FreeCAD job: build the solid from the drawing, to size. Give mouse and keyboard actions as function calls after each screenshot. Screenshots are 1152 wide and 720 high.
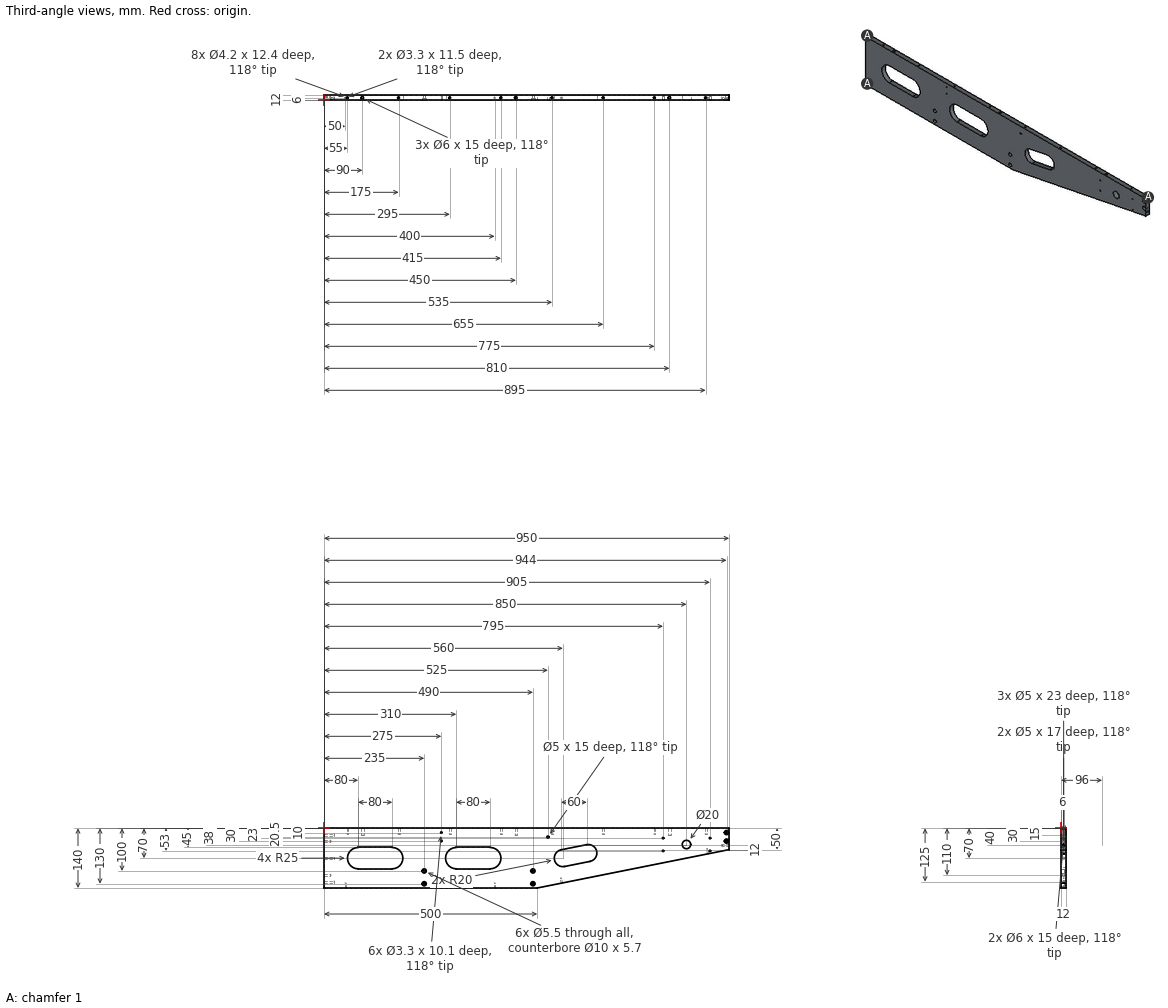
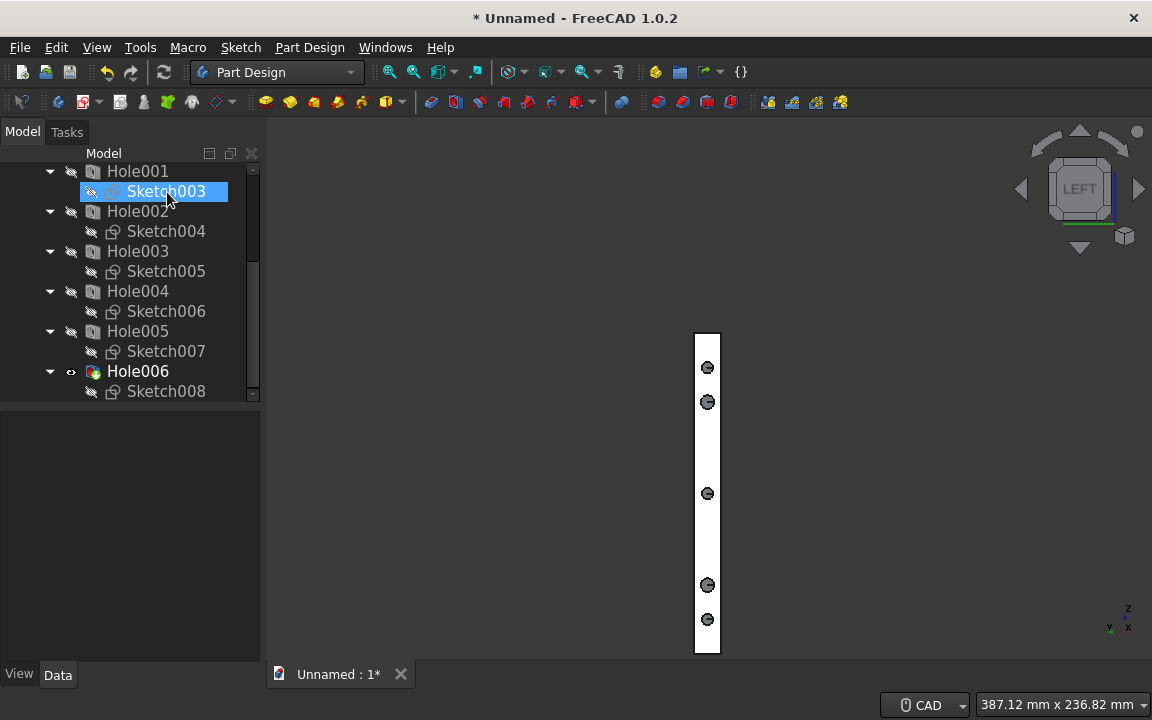
click(84, 102)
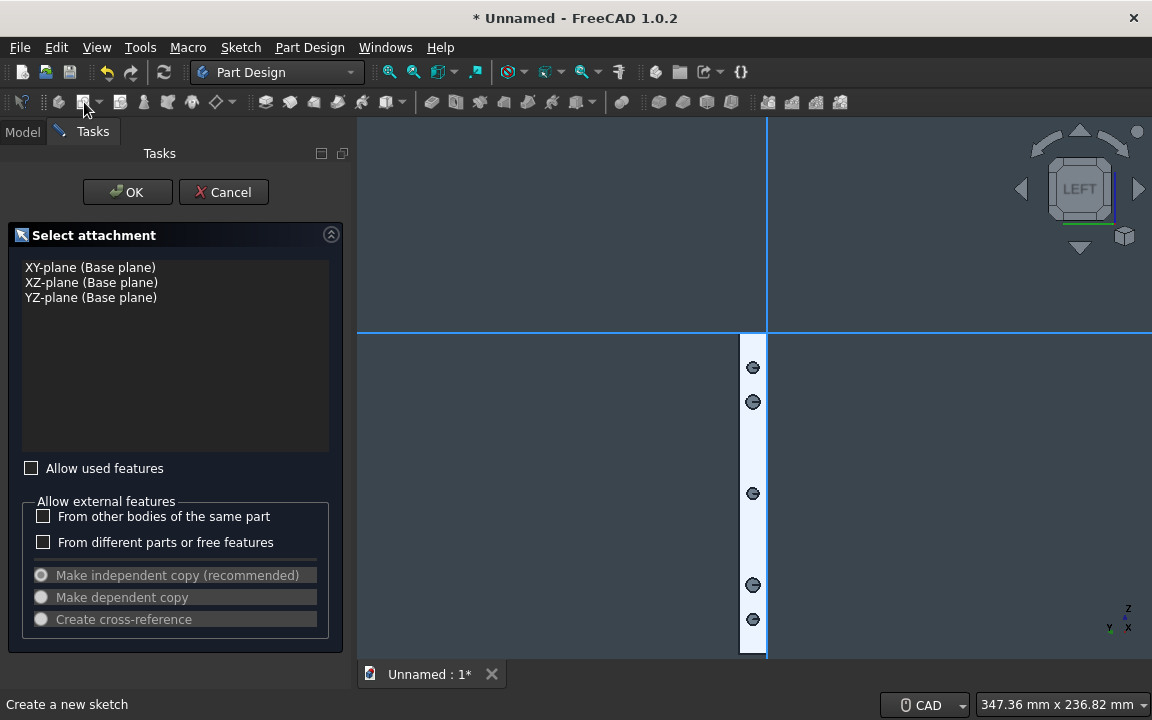
click(82, 268)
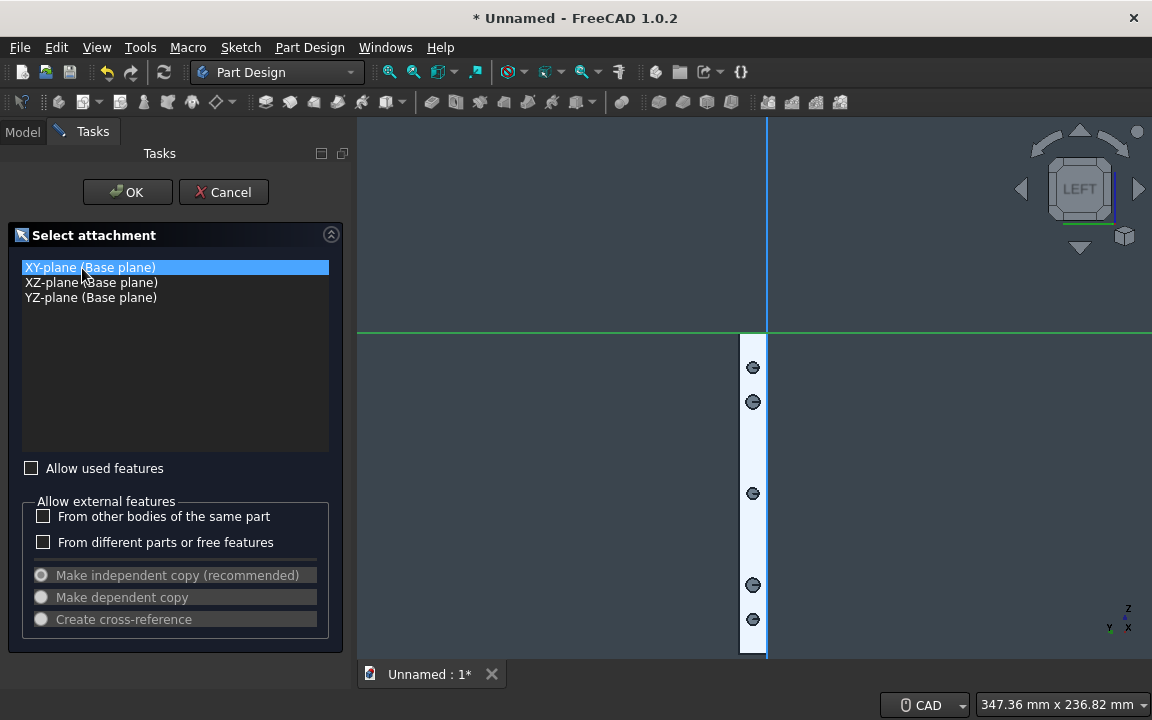
click(128, 192)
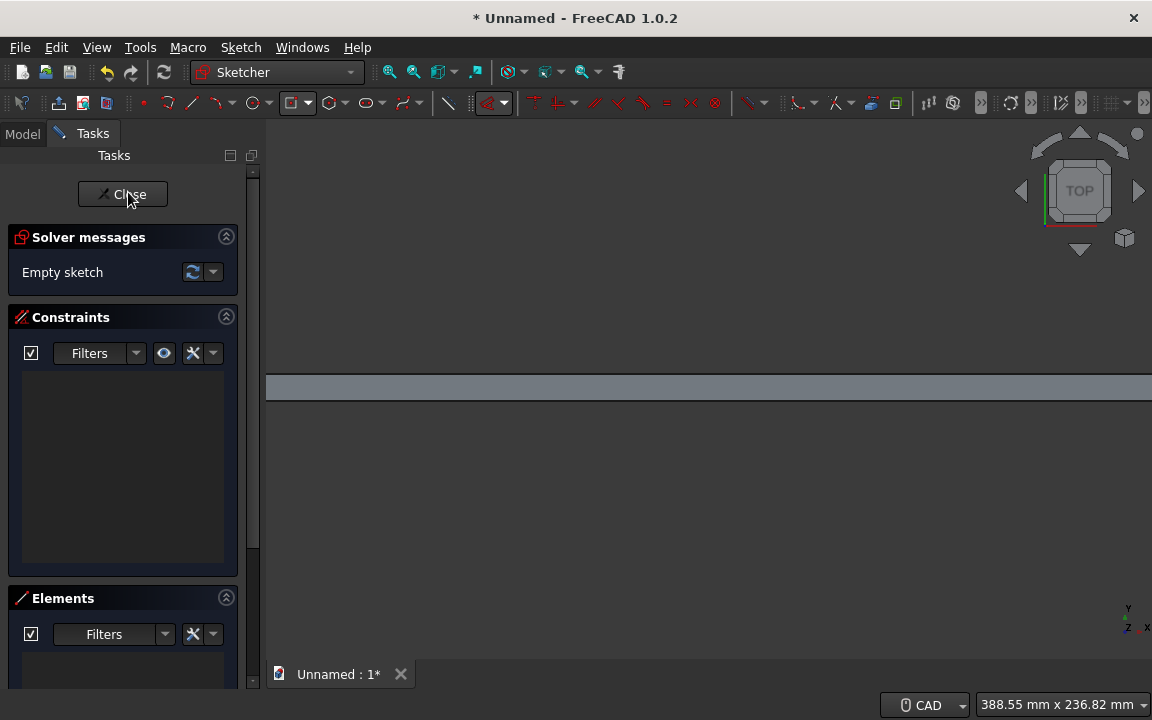
scroll(638, 388, down, 7)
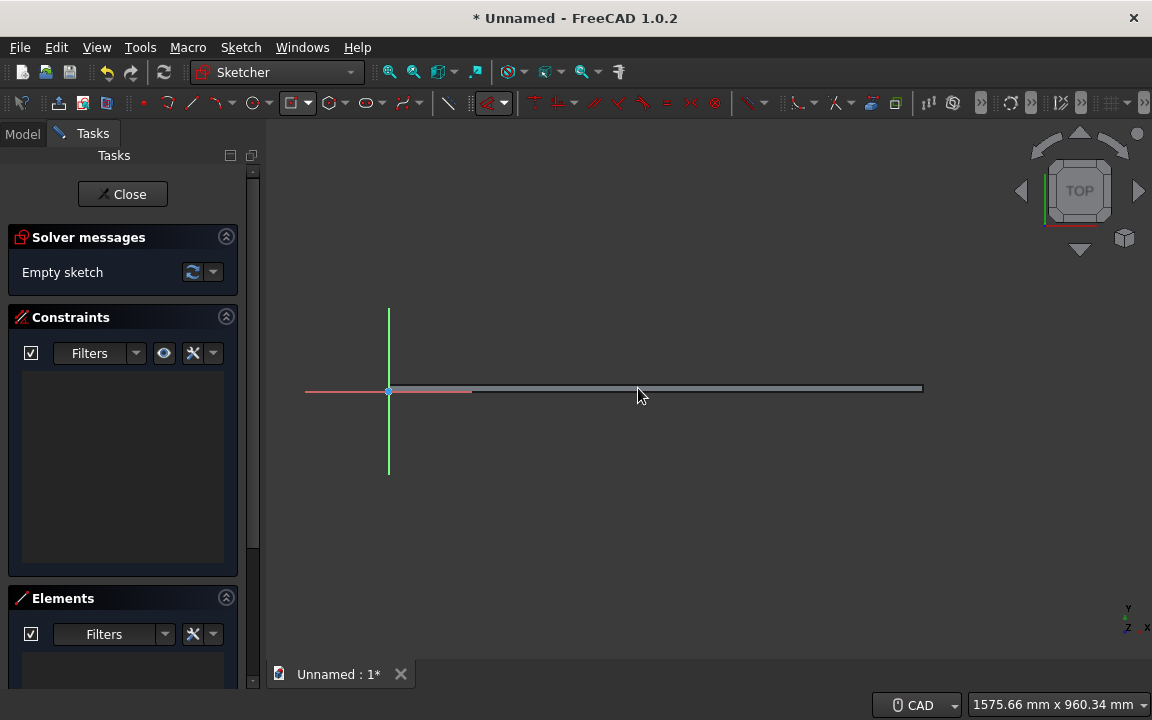
key(g)
key(c)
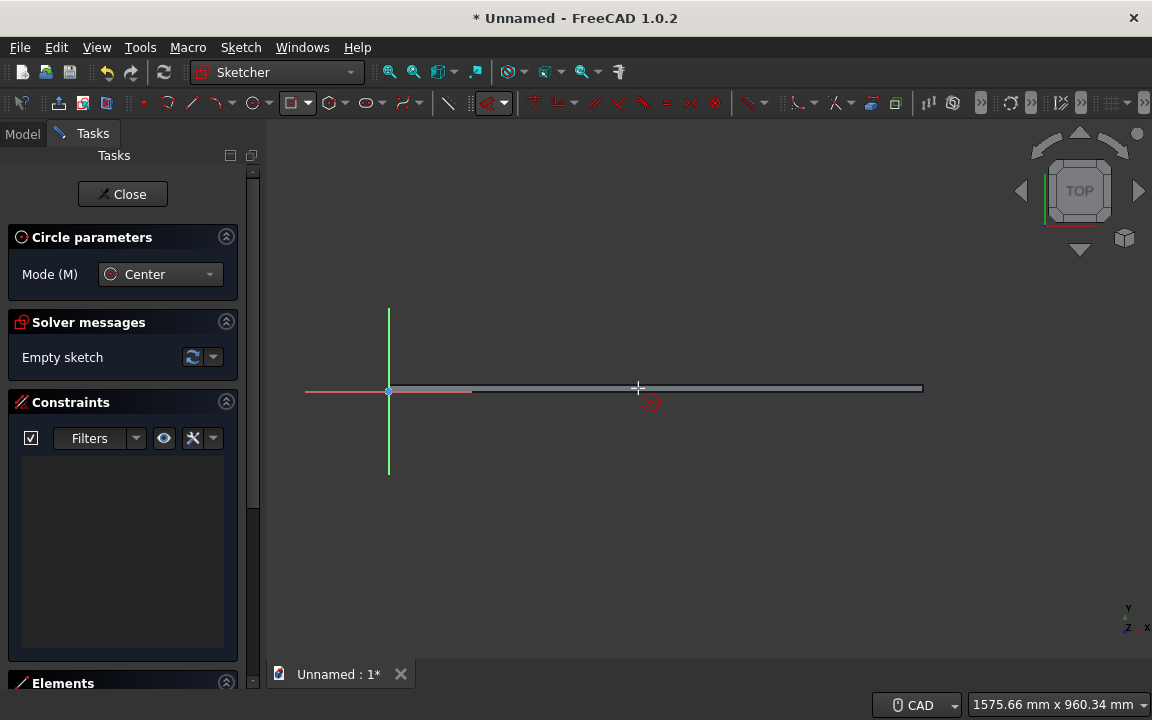
scroll(420, 388, up, 15)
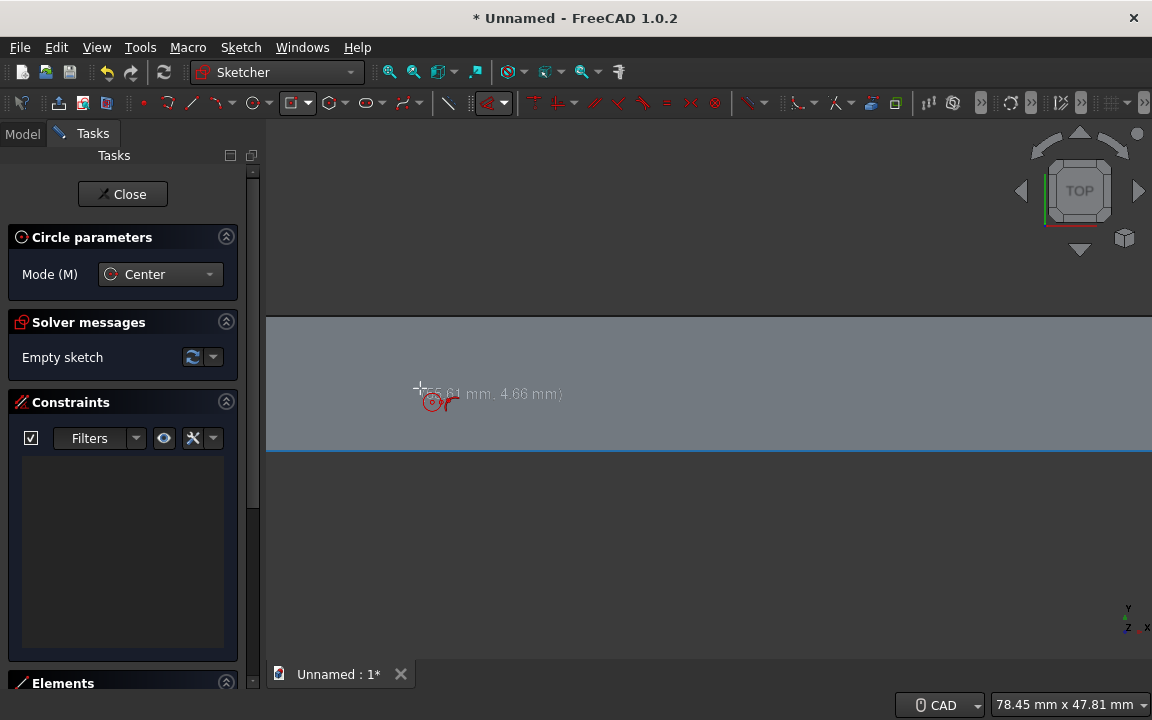
scroll(420, 388, down, 15)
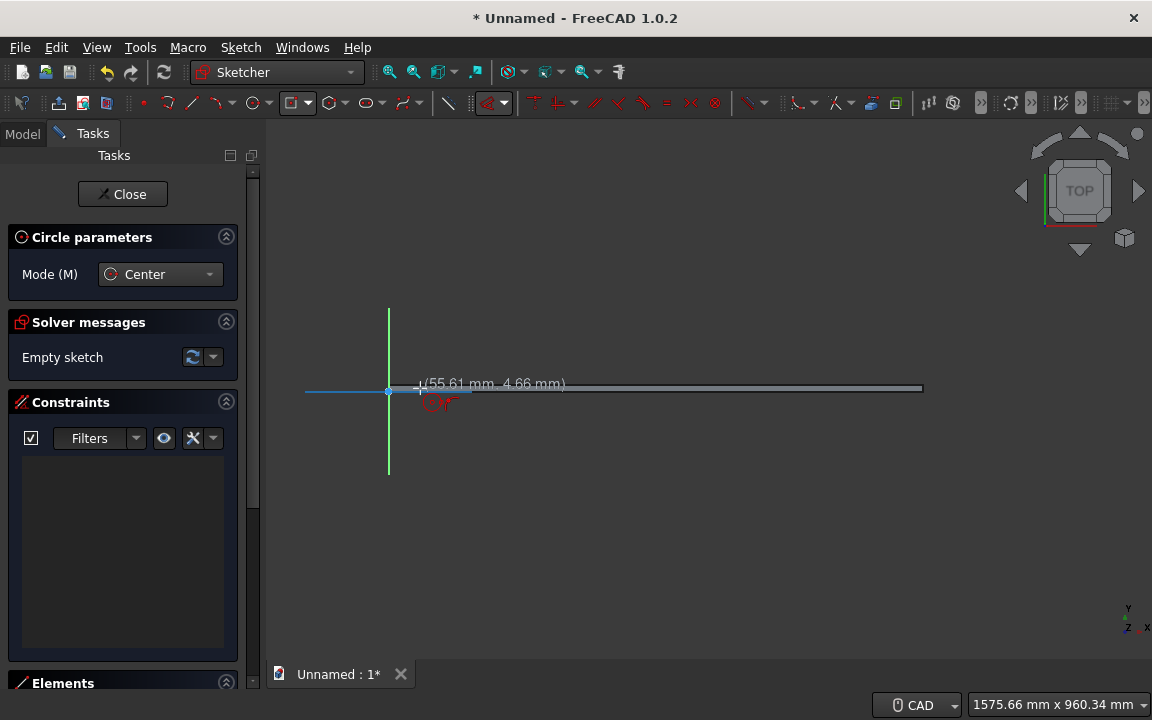
scroll(420, 388, up, 8)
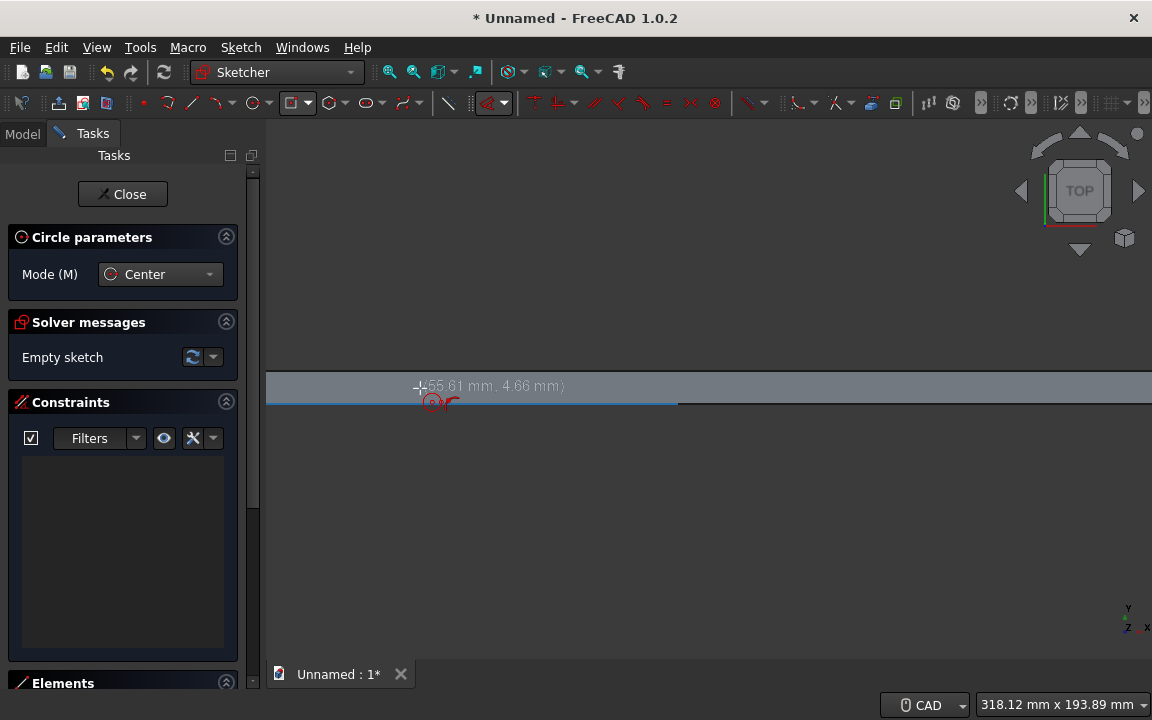
click(418, 387)
move(422, 383)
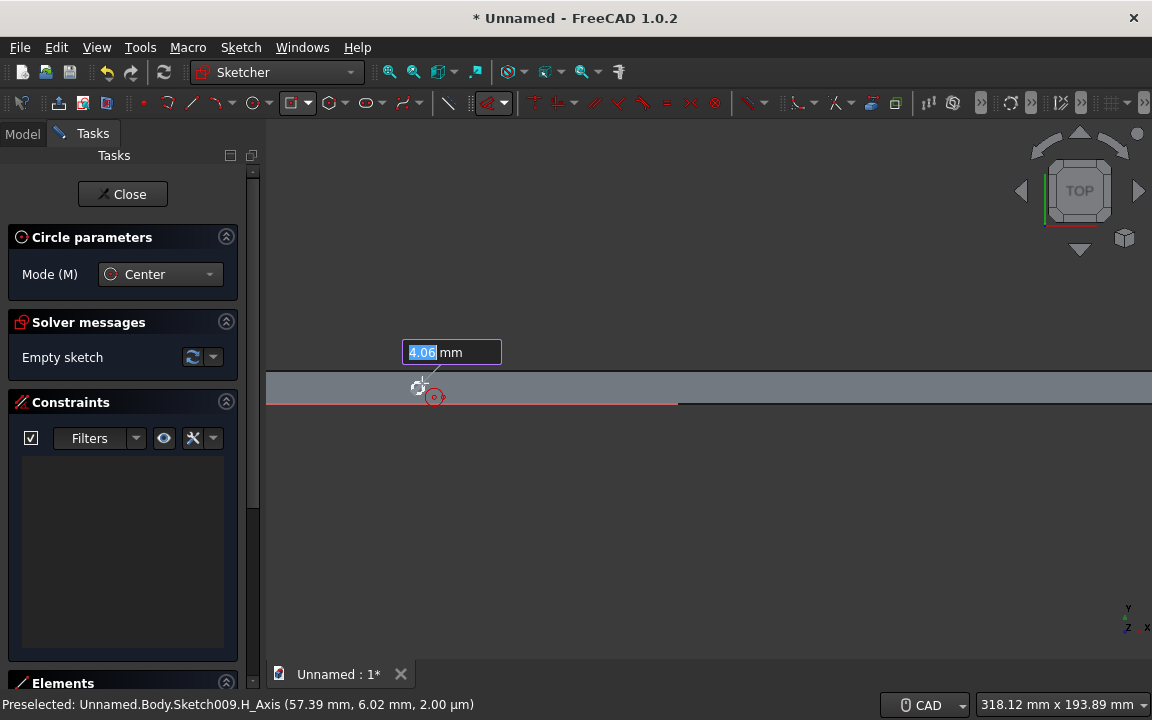
text(4.2)
key(Return)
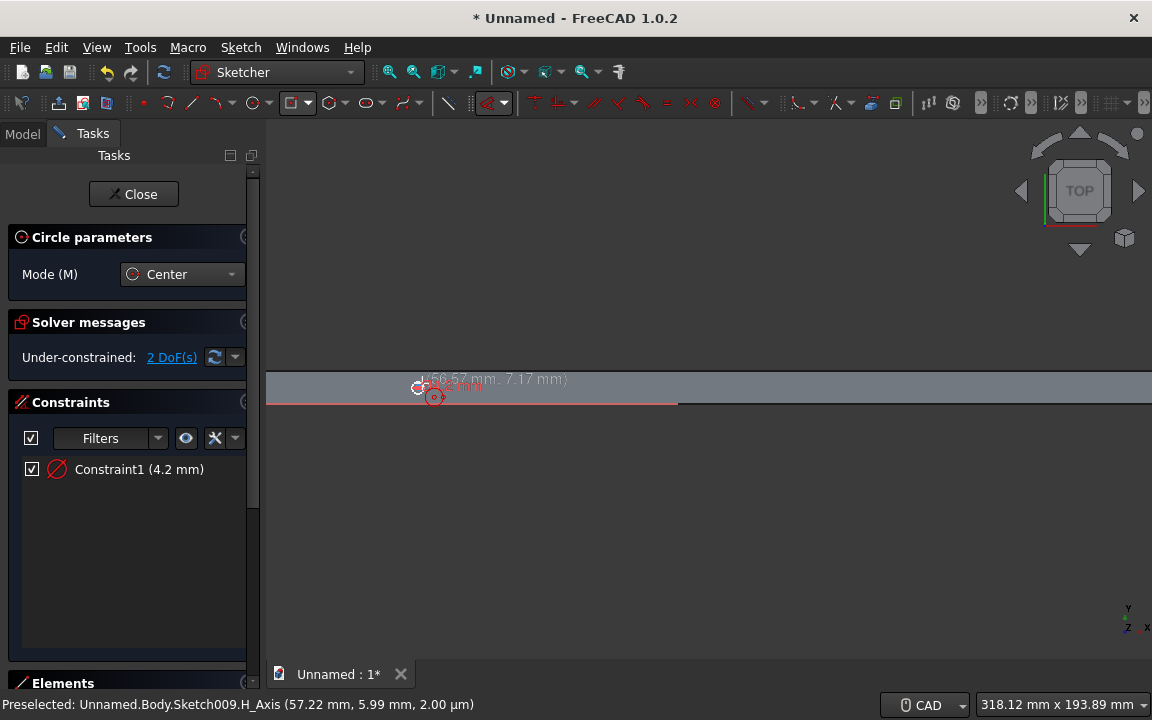
scroll(752, 387, up, 7)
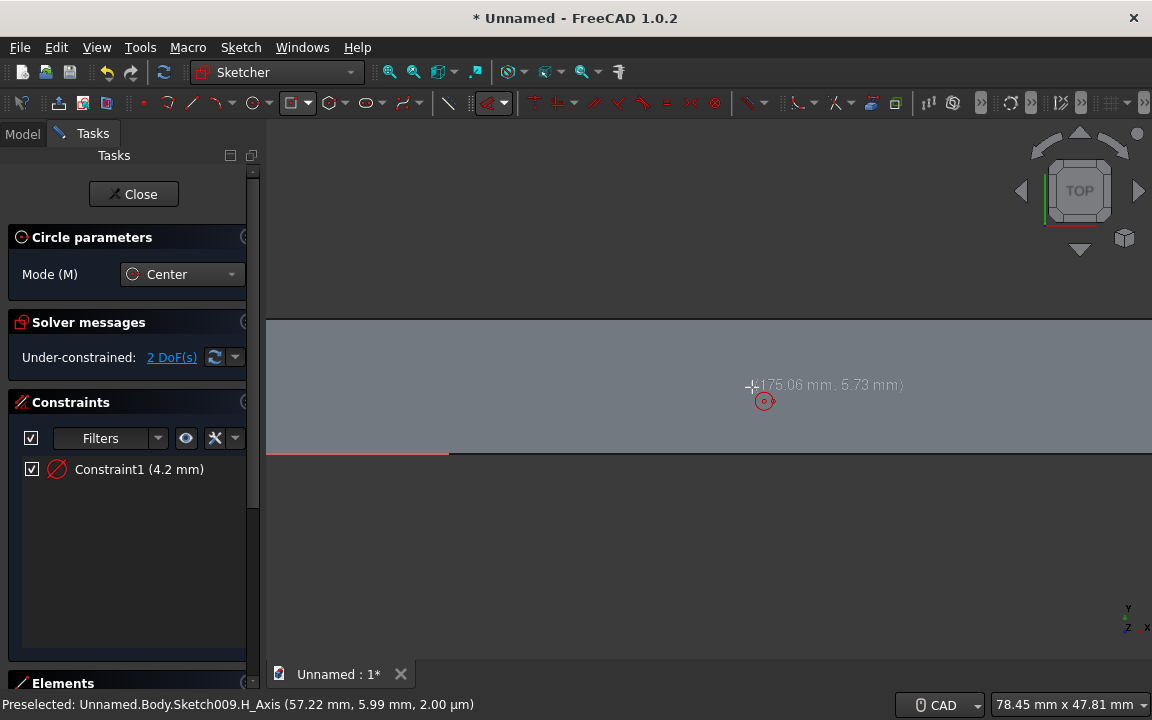
scroll(473, 388, down, 15)